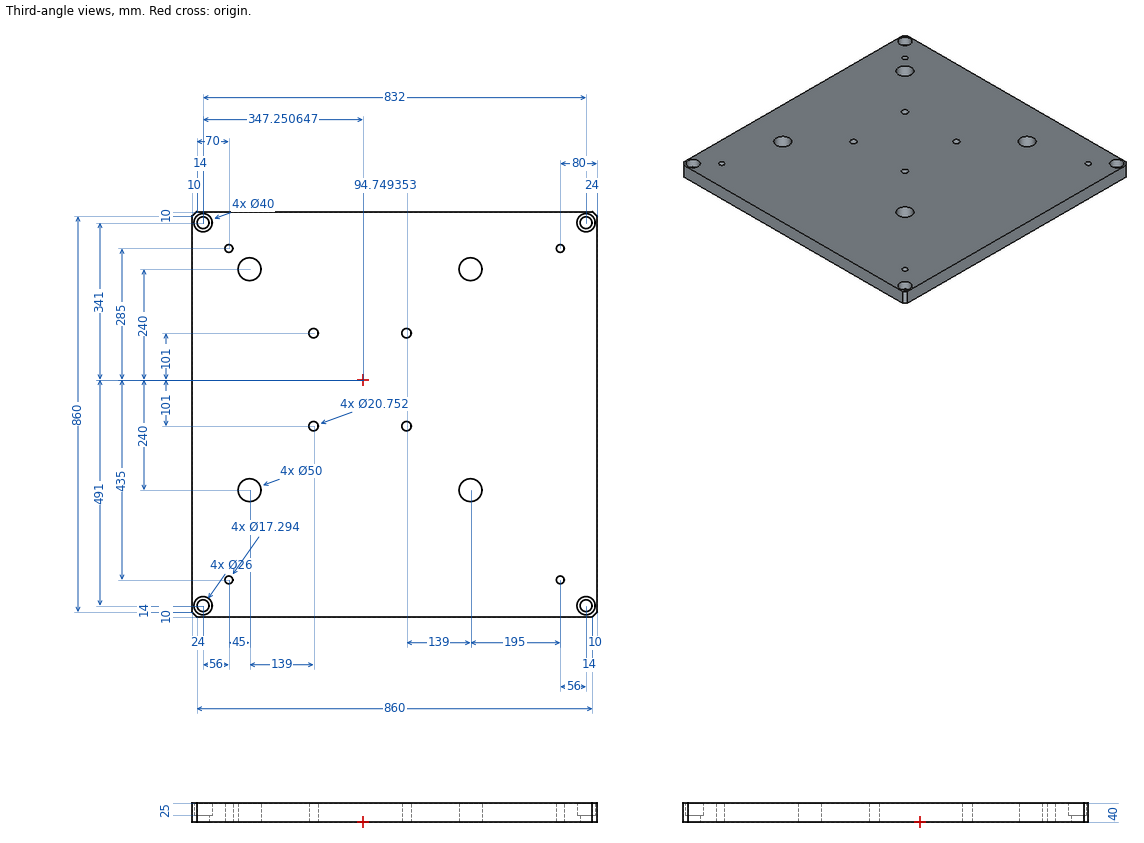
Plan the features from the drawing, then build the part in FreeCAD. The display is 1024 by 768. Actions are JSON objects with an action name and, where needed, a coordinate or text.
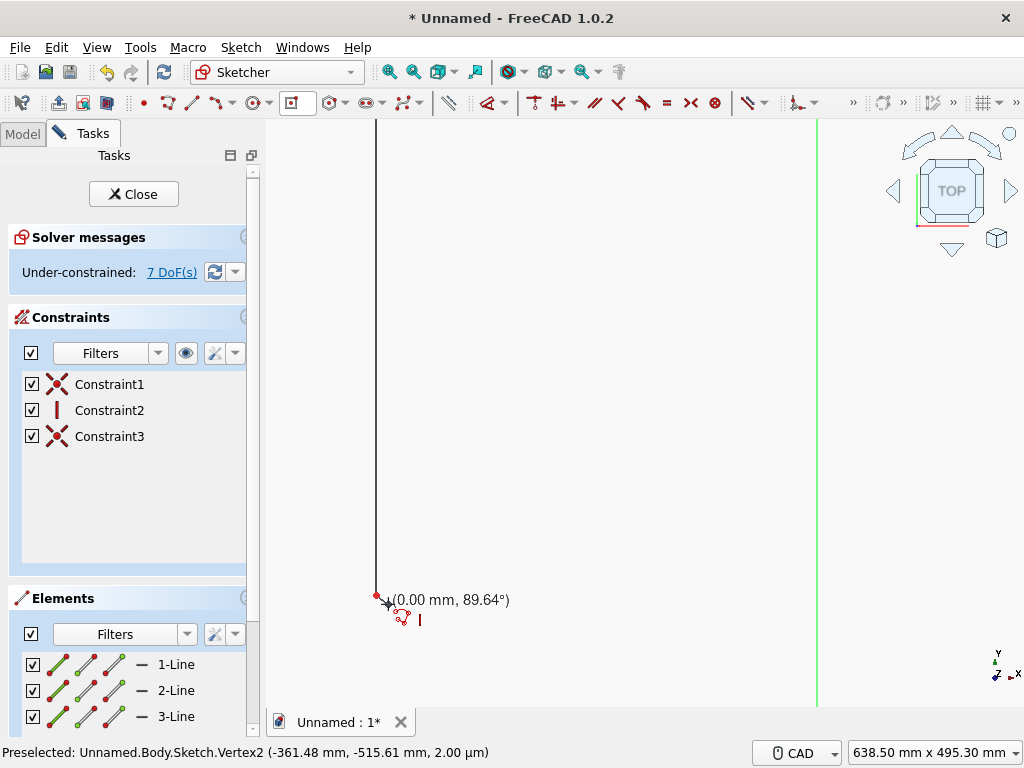
{"action": "scroll", "coordinate": [389, 606], "scroll_direction": "down", "scroll_amount": 5}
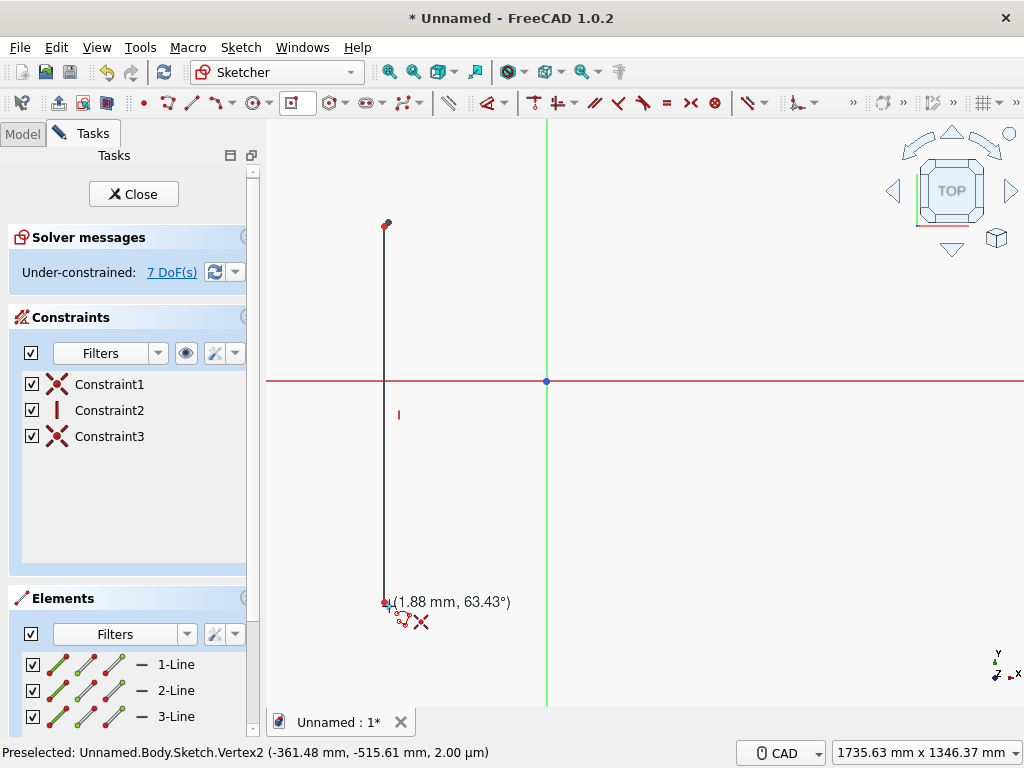
{"action": "left_click", "coordinate": [764, 606]}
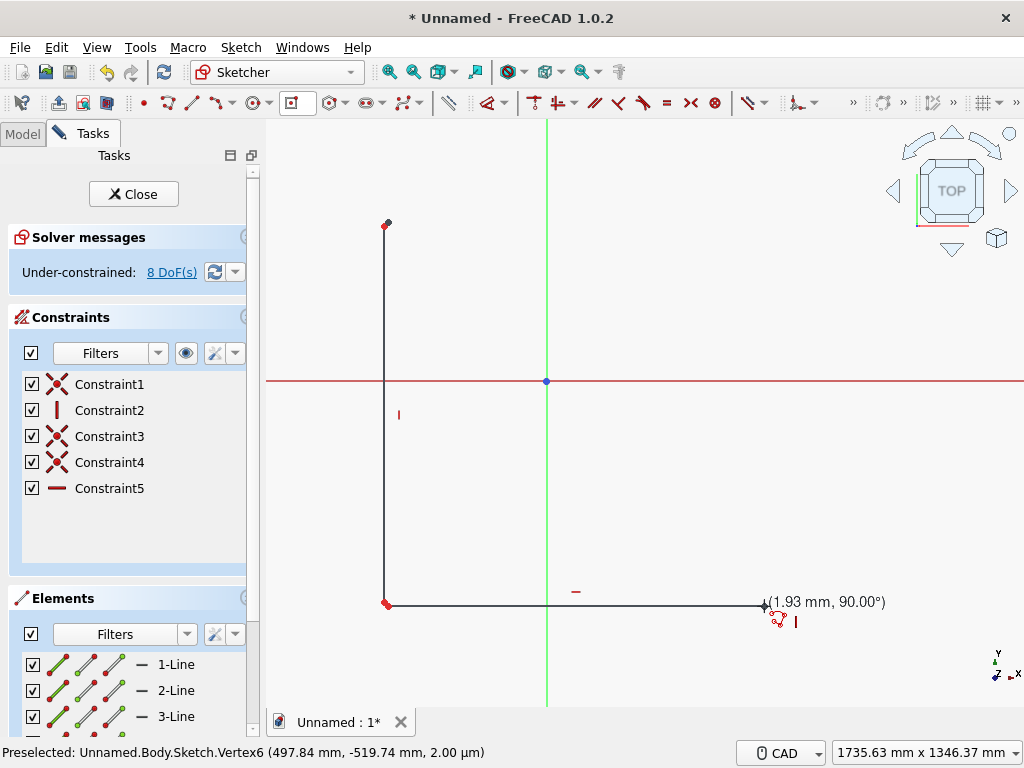
{"action": "scroll", "coordinate": [769, 602], "scroll_direction": "up", "scroll_amount": 5}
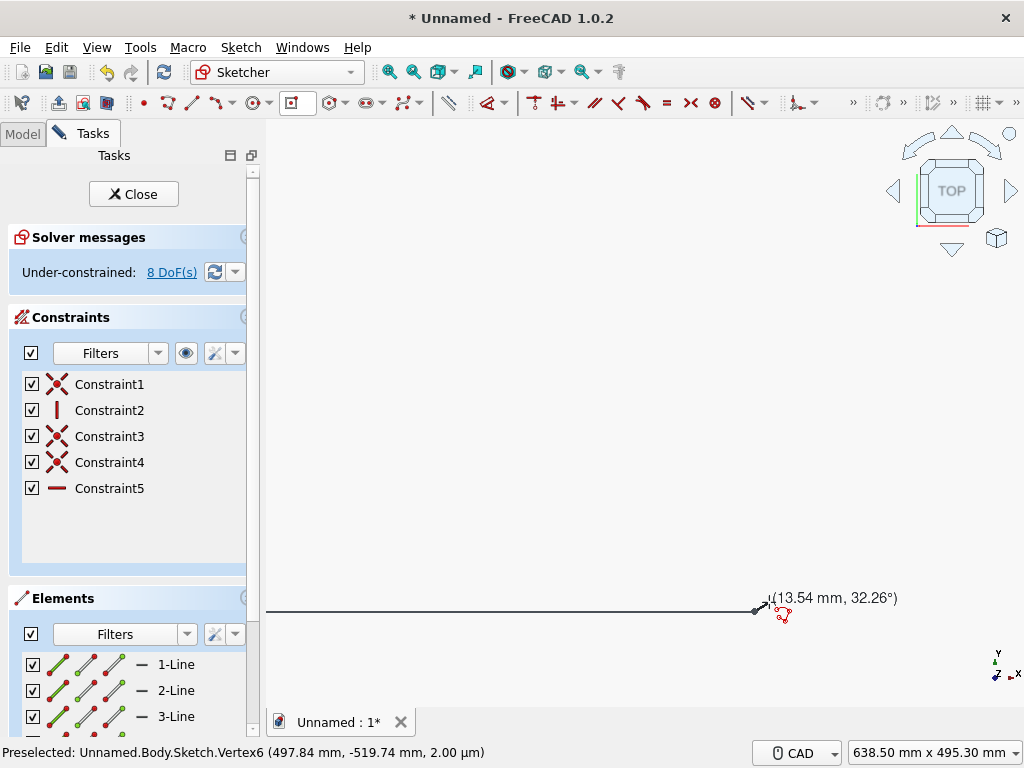
{"action": "left_click", "coordinate": [767, 599]}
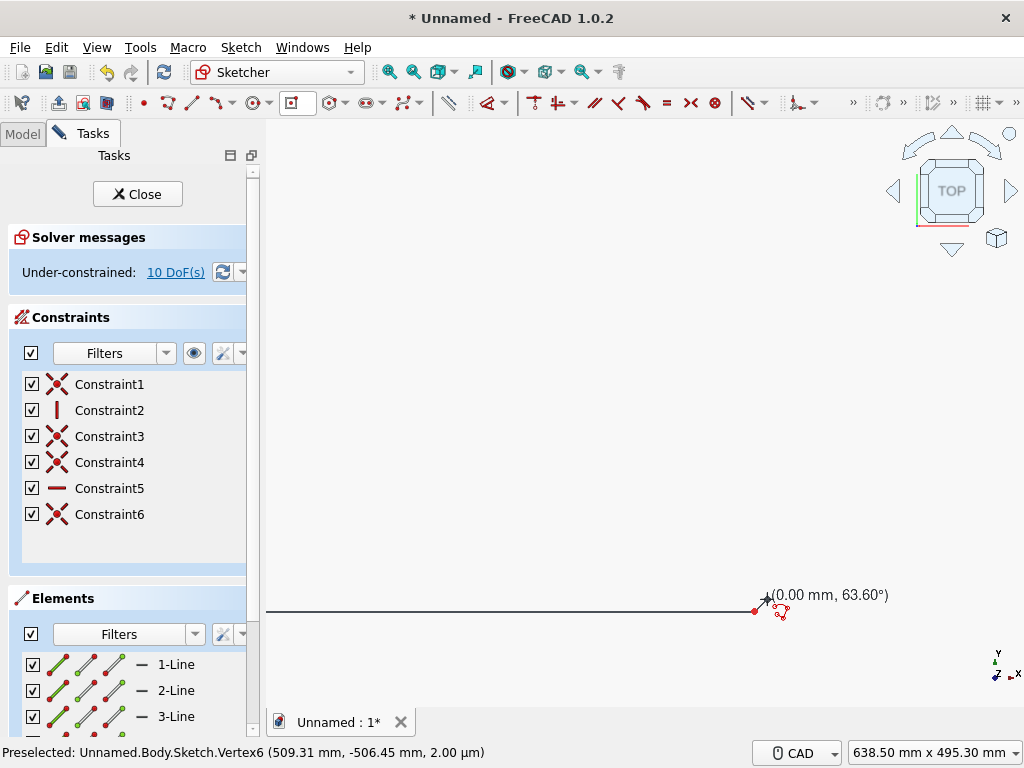
{"action": "scroll", "coordinate": [770, 602], "scroll_direction": "down", "scroll_amount": 5}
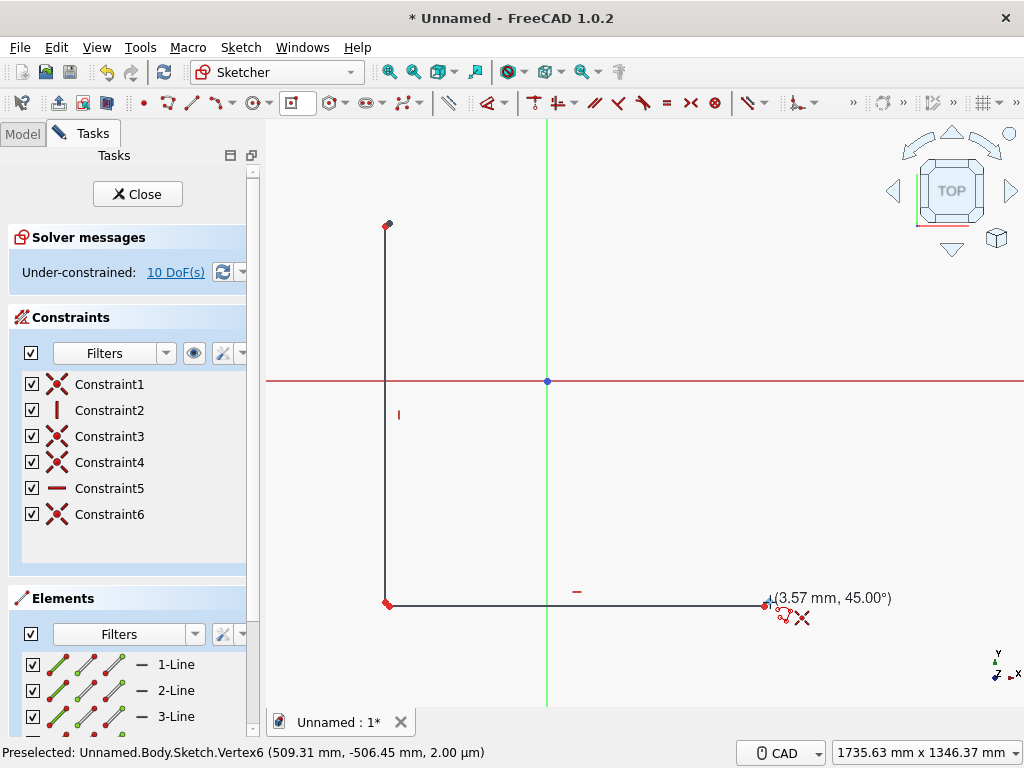
{"action": "left_click", "coordinate": [769, 226]}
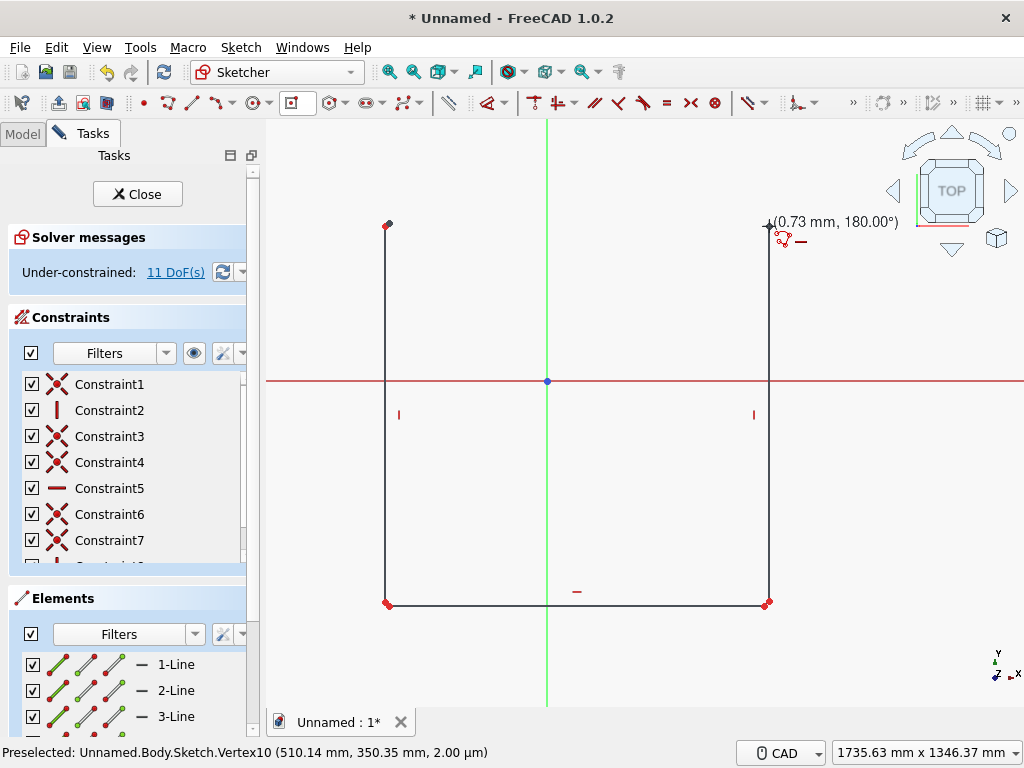
{"action": "scroll", "coordinate": [765, 222], "scroll_direction": "up", "scroll_amount": 5}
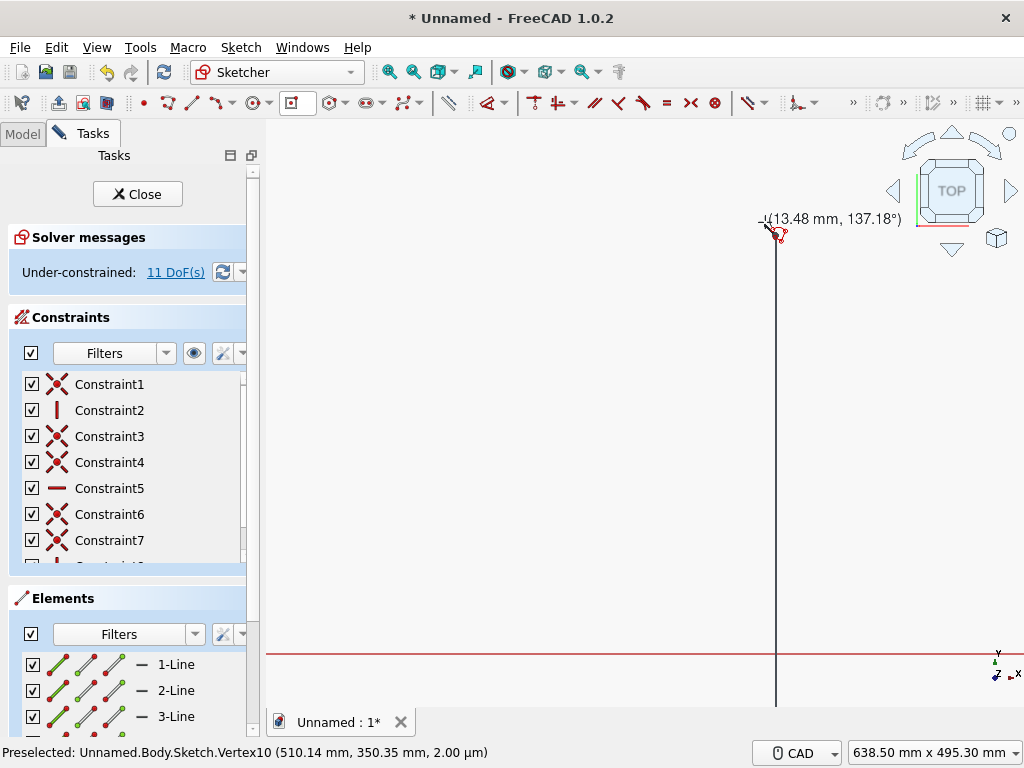
{"action": "left_click", "coordinate": [764, 221]}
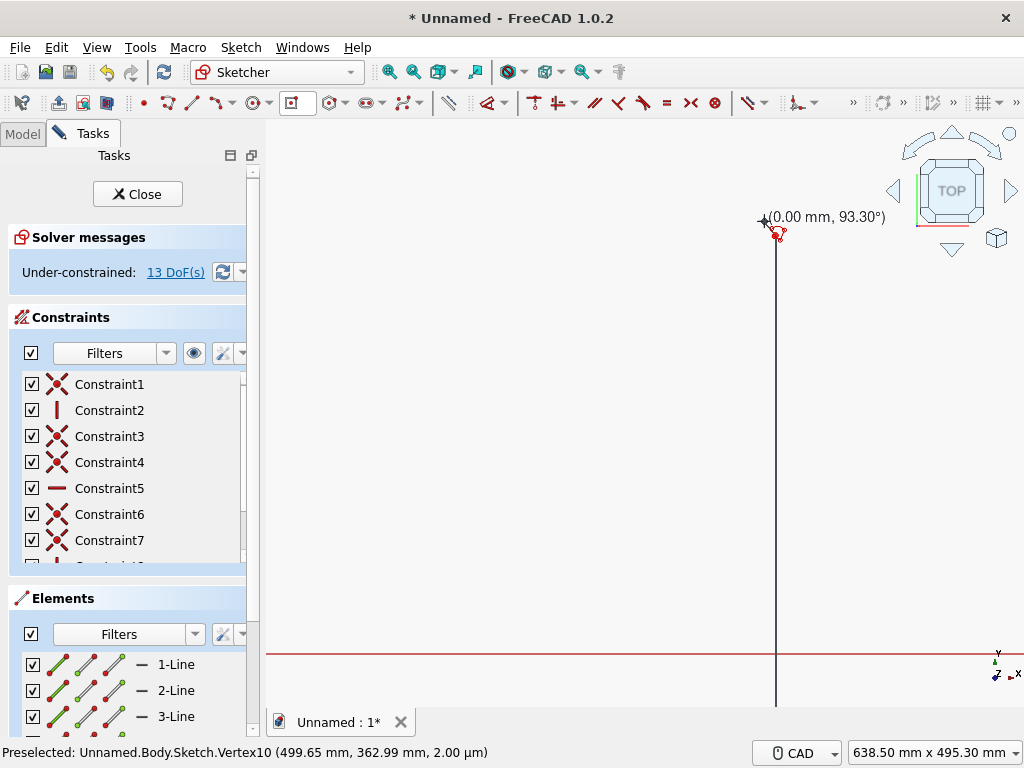
{"action": "scroll", "coordinate": [765, 221], "scroll_direction": "down", "scroll_amount": 5}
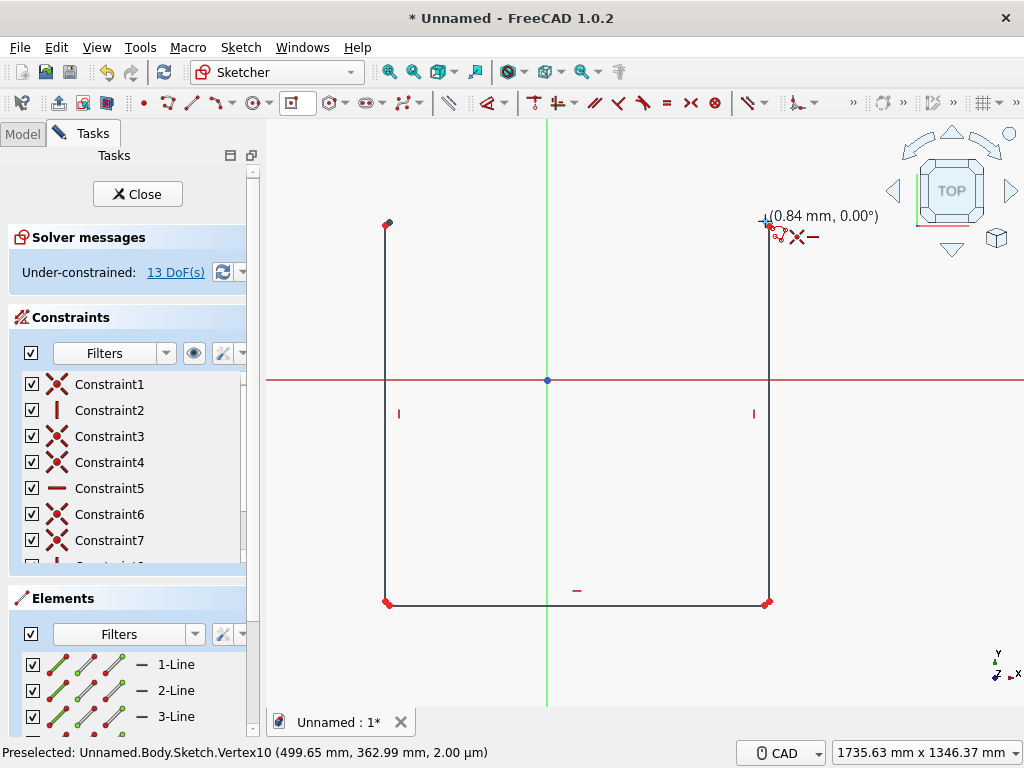
{"action": "scroll", "coordinate": [389, 221], "scroll_direction": "up", "scroll_amount": 9}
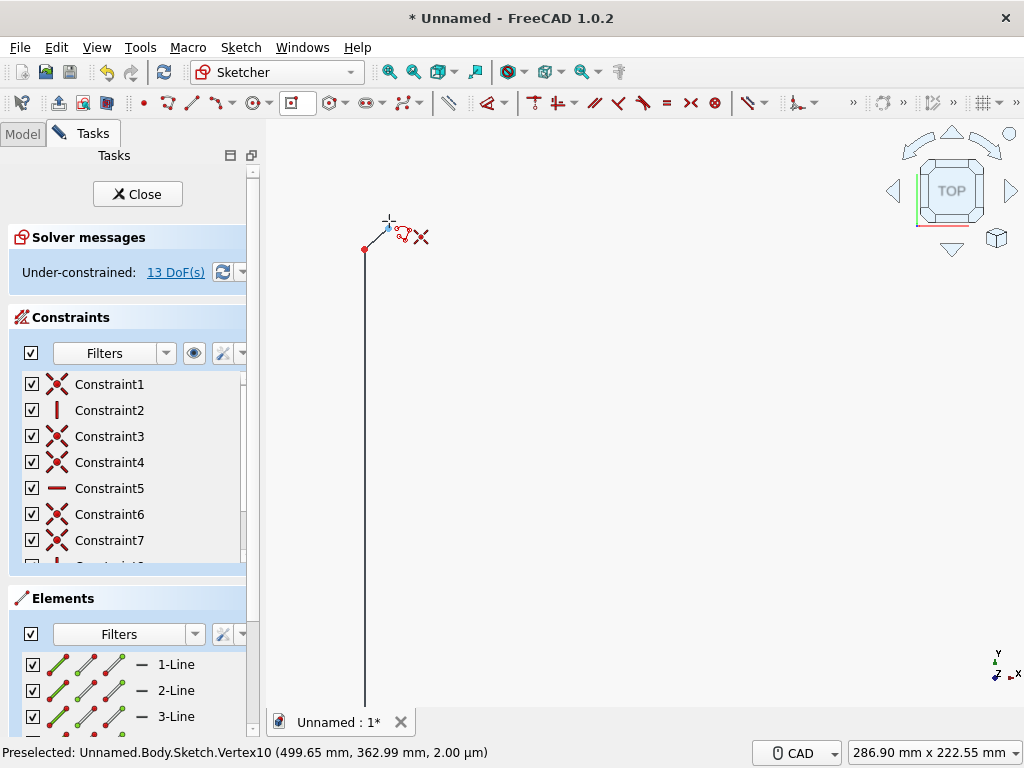
{"action": "left_click", "coordinate": [388, 228]}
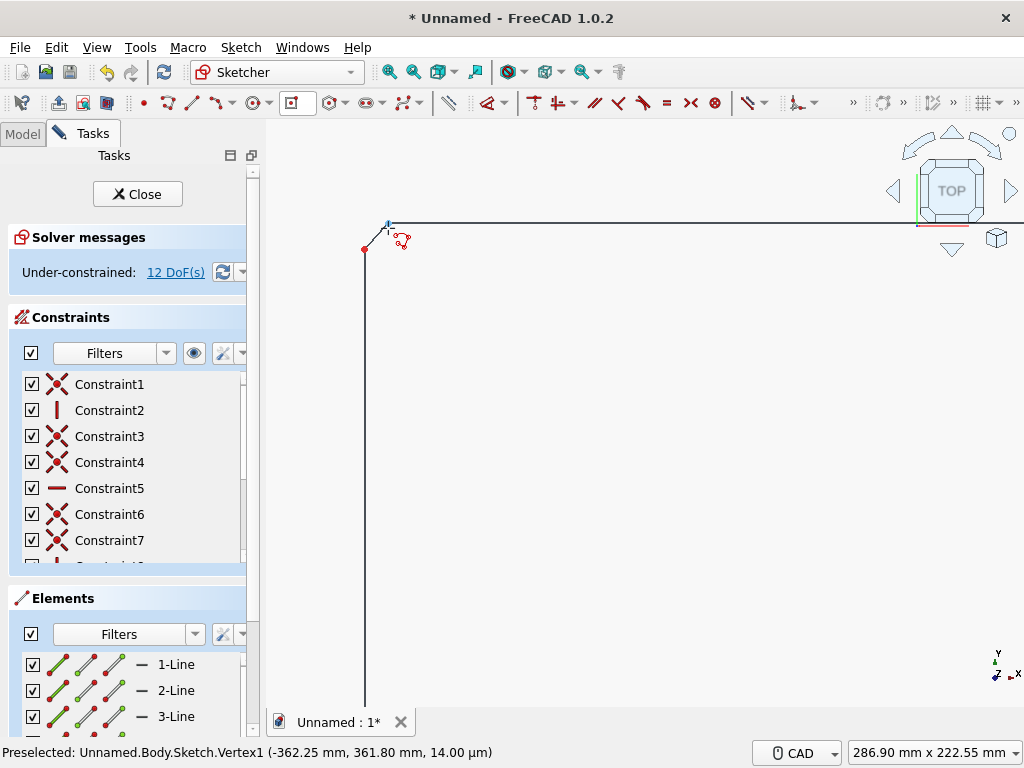
{"action": "key", "text": "g c"}